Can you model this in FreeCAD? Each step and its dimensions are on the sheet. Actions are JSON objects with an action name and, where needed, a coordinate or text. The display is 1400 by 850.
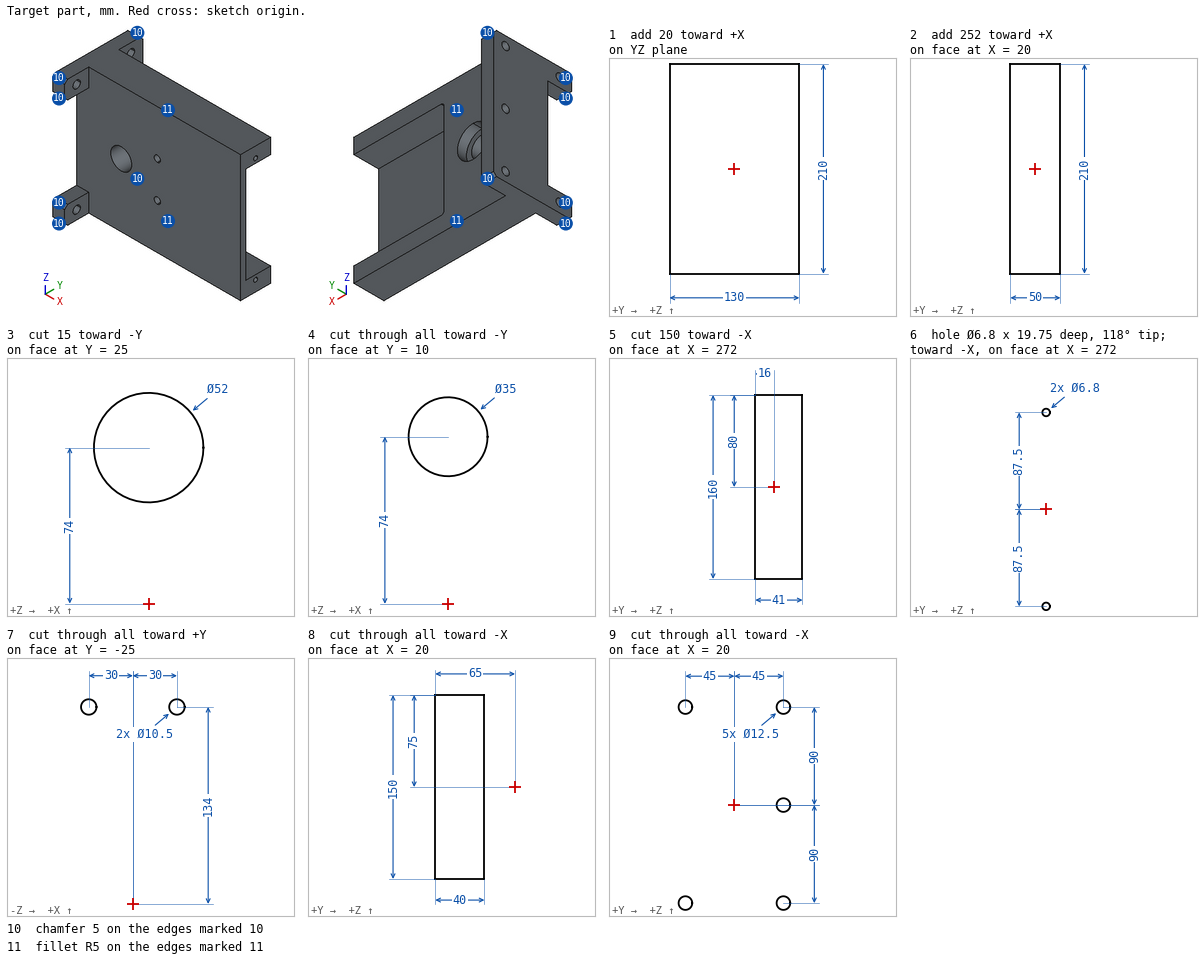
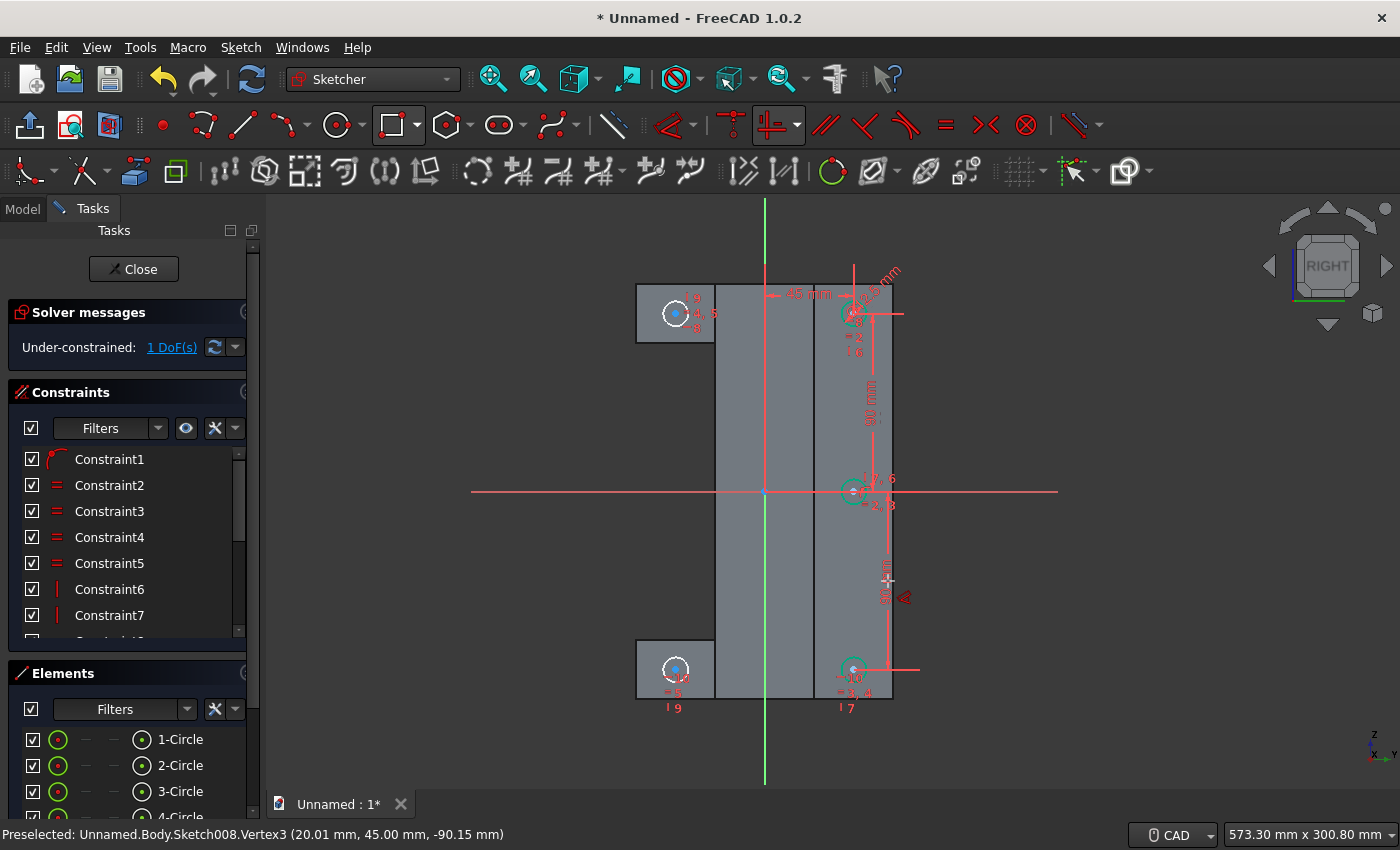
{"action": "left_click", "coordinate": [676, 314]}
{"action": "left_click", "coordinate": [720, 280]}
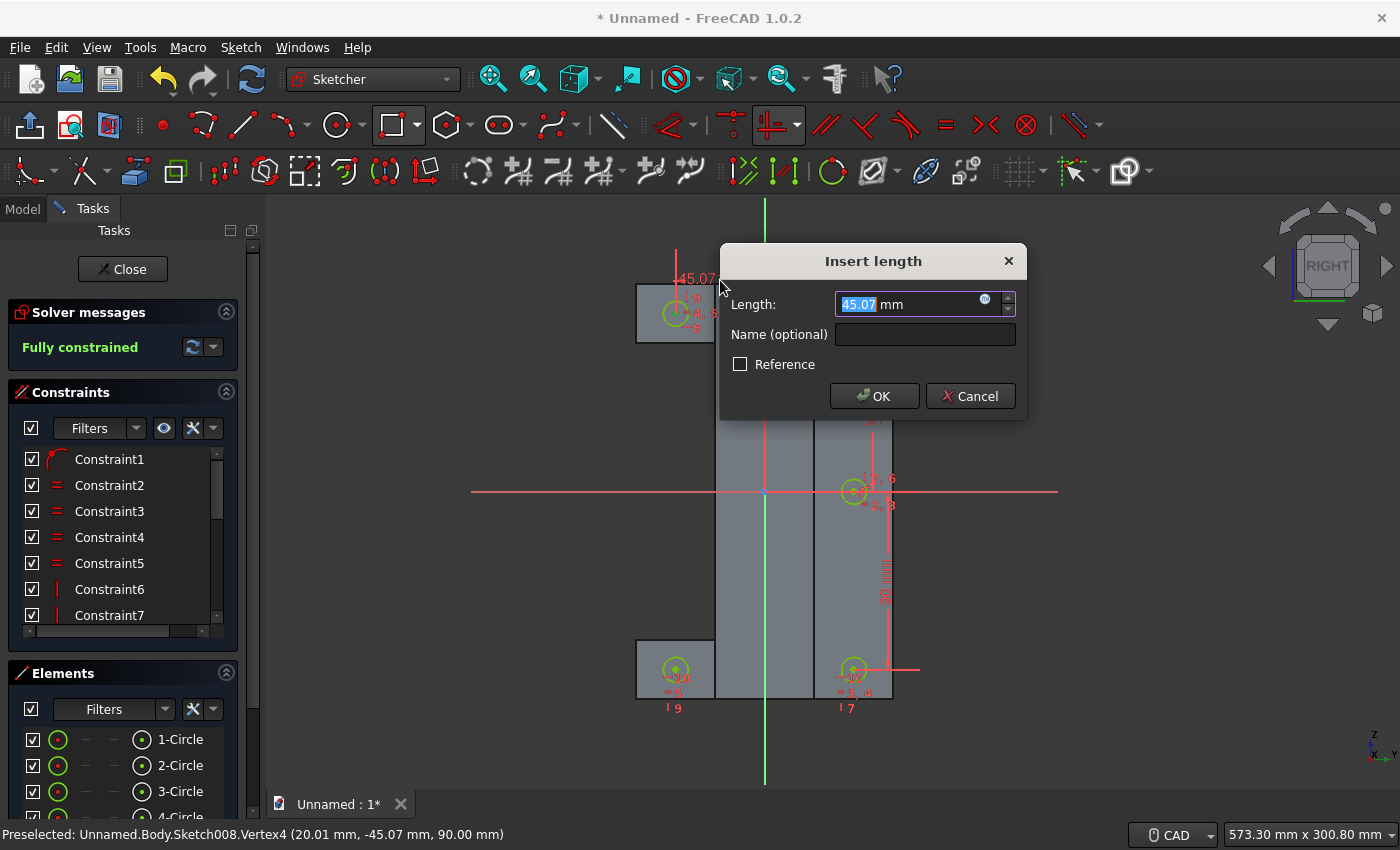
{"action": "type", "text": "45"}
{"action": "key", "text": "Return"}
{"action": "key", "text": "Escape"}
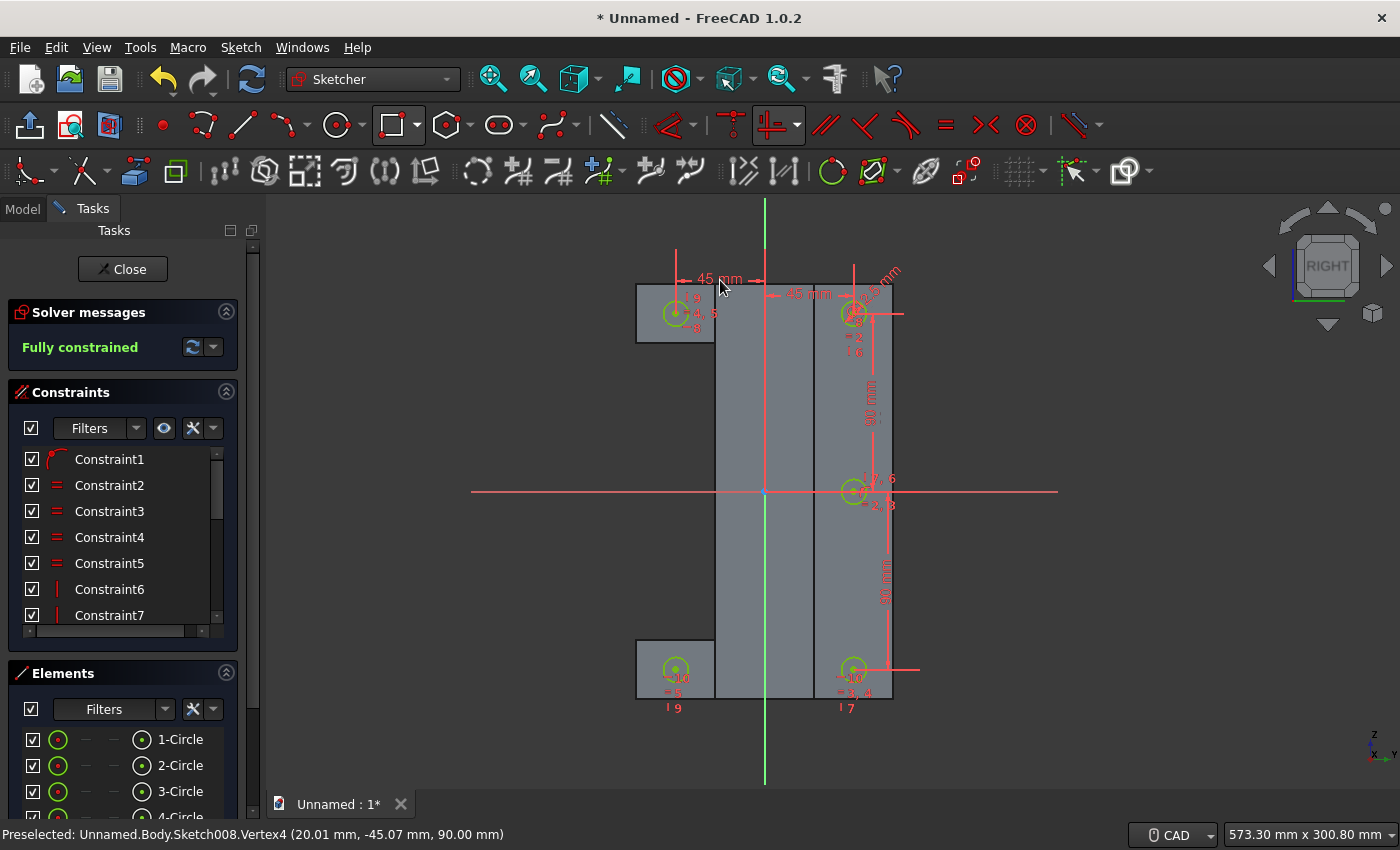
{"action": "left_click", "coordinate": [123, 269]}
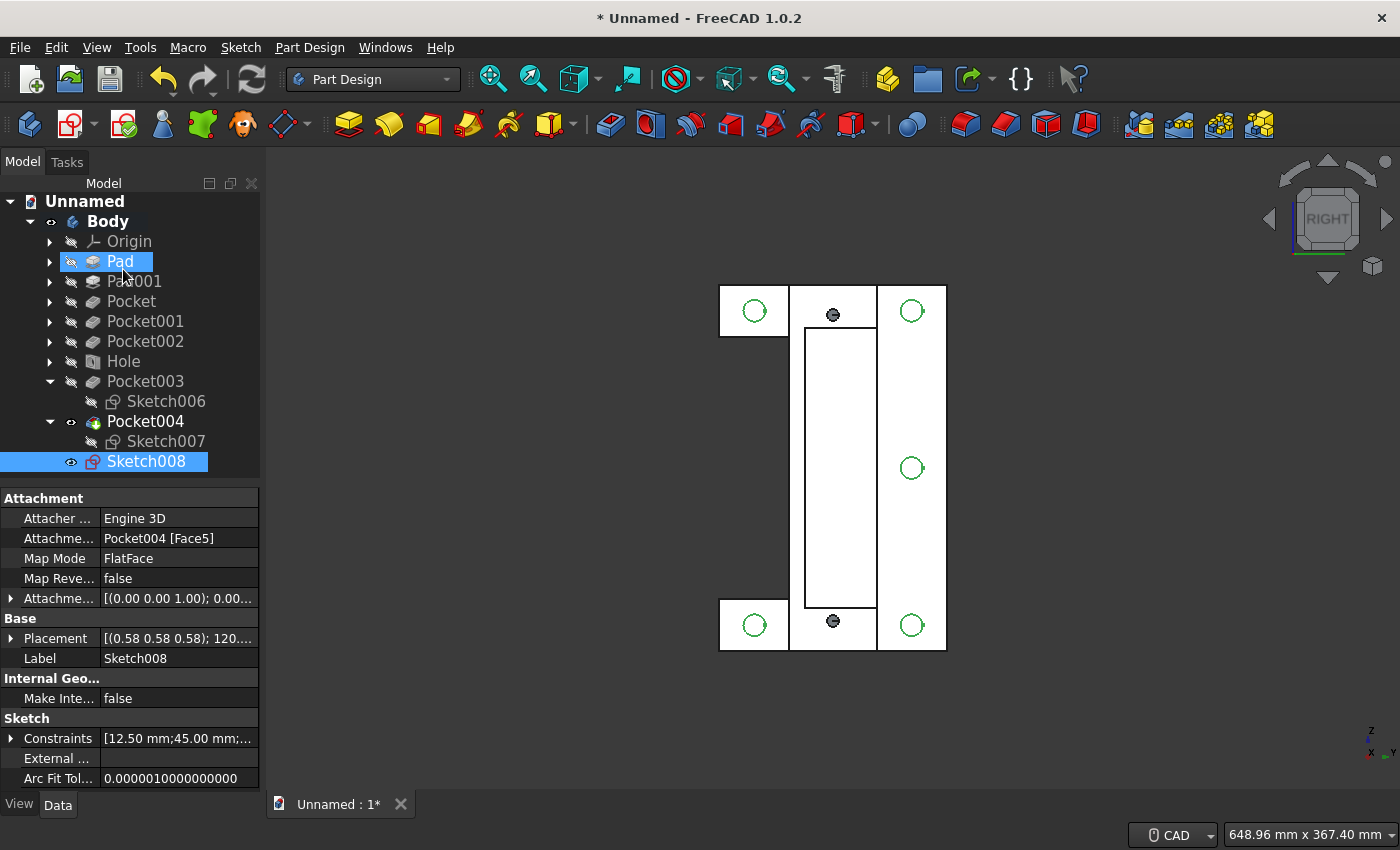
{"action": "left_click", "coordinate": [612, 124]}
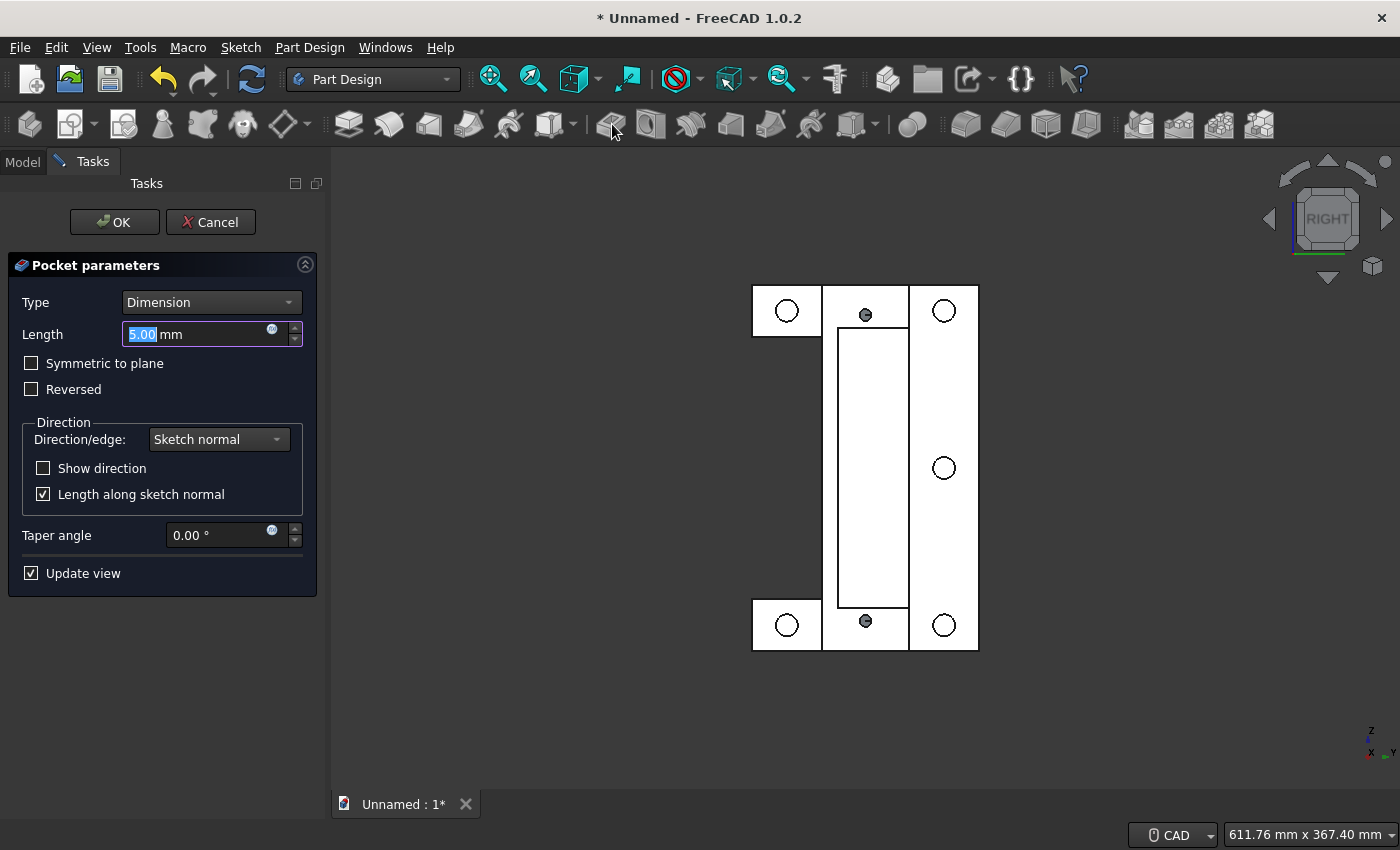
{"action": "left_click", "coordinate": [212, 302]}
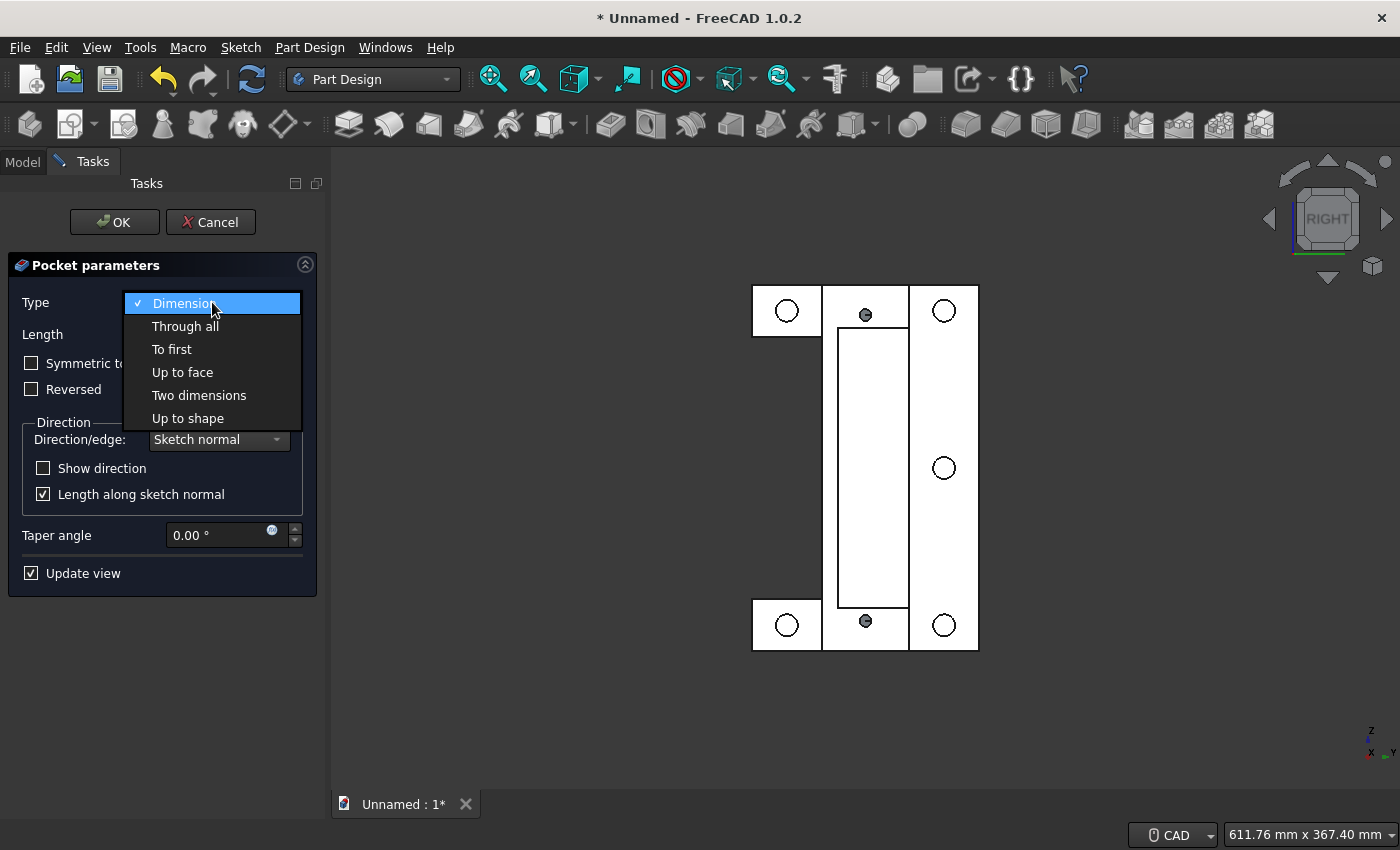
{"action": "left_click", "coordinate": [212, 326]}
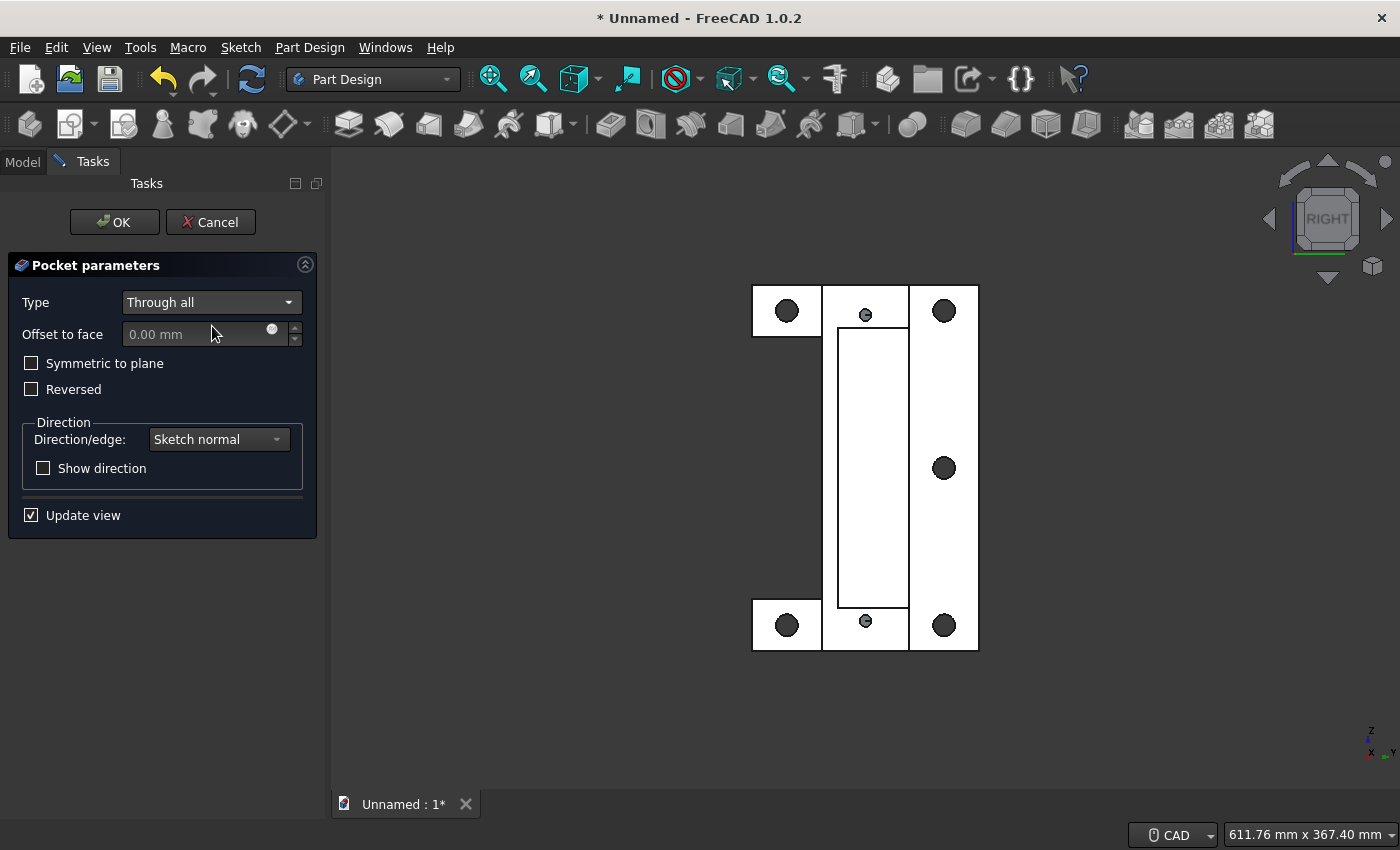
{"action": "left_click", "coordinate": [115, 222]}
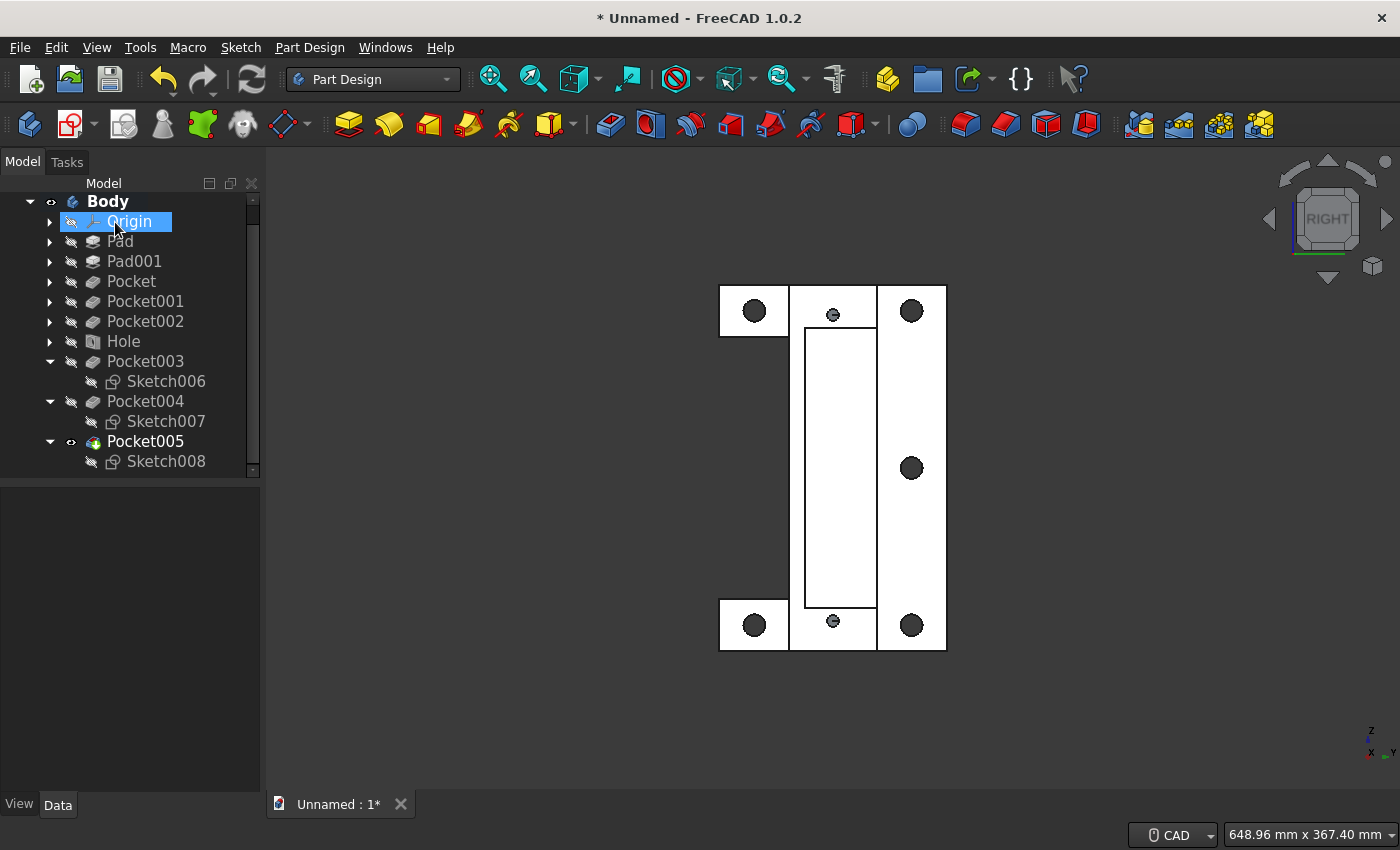
{"action": "key", "text": "0"}